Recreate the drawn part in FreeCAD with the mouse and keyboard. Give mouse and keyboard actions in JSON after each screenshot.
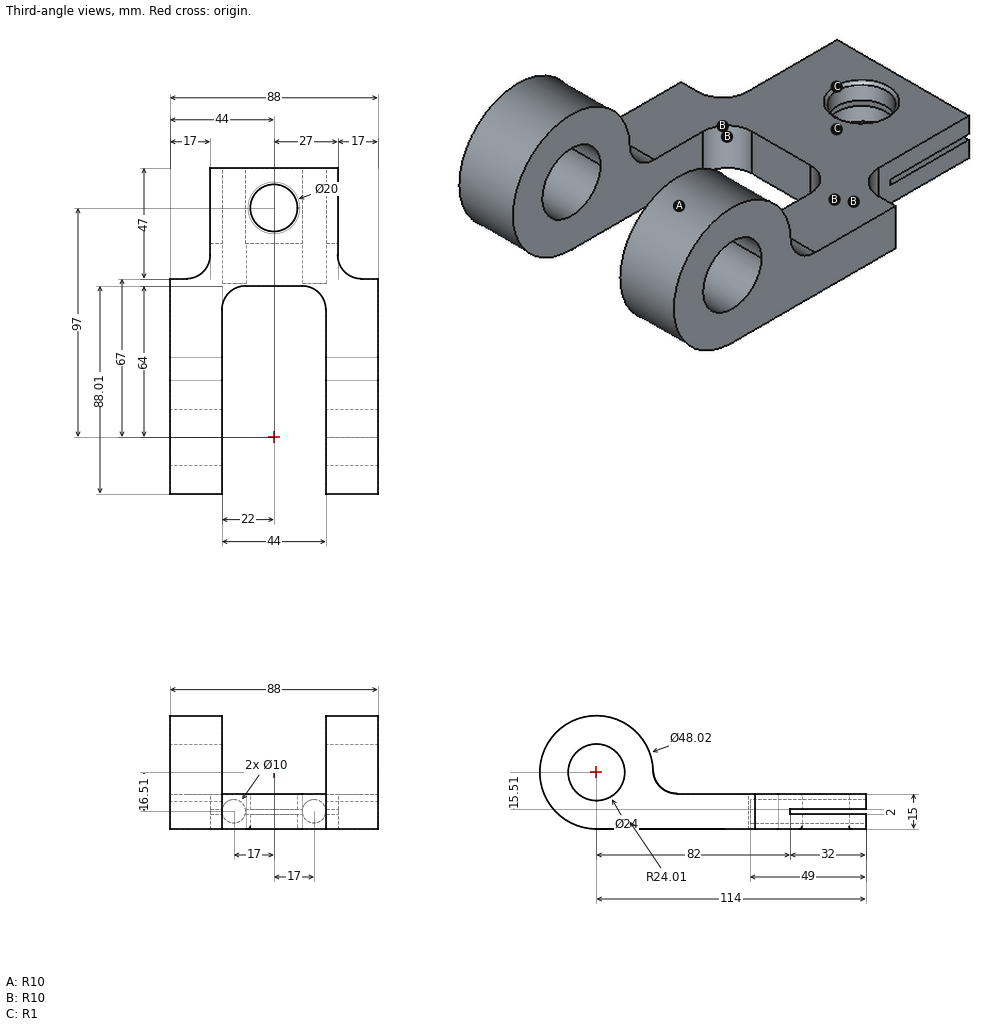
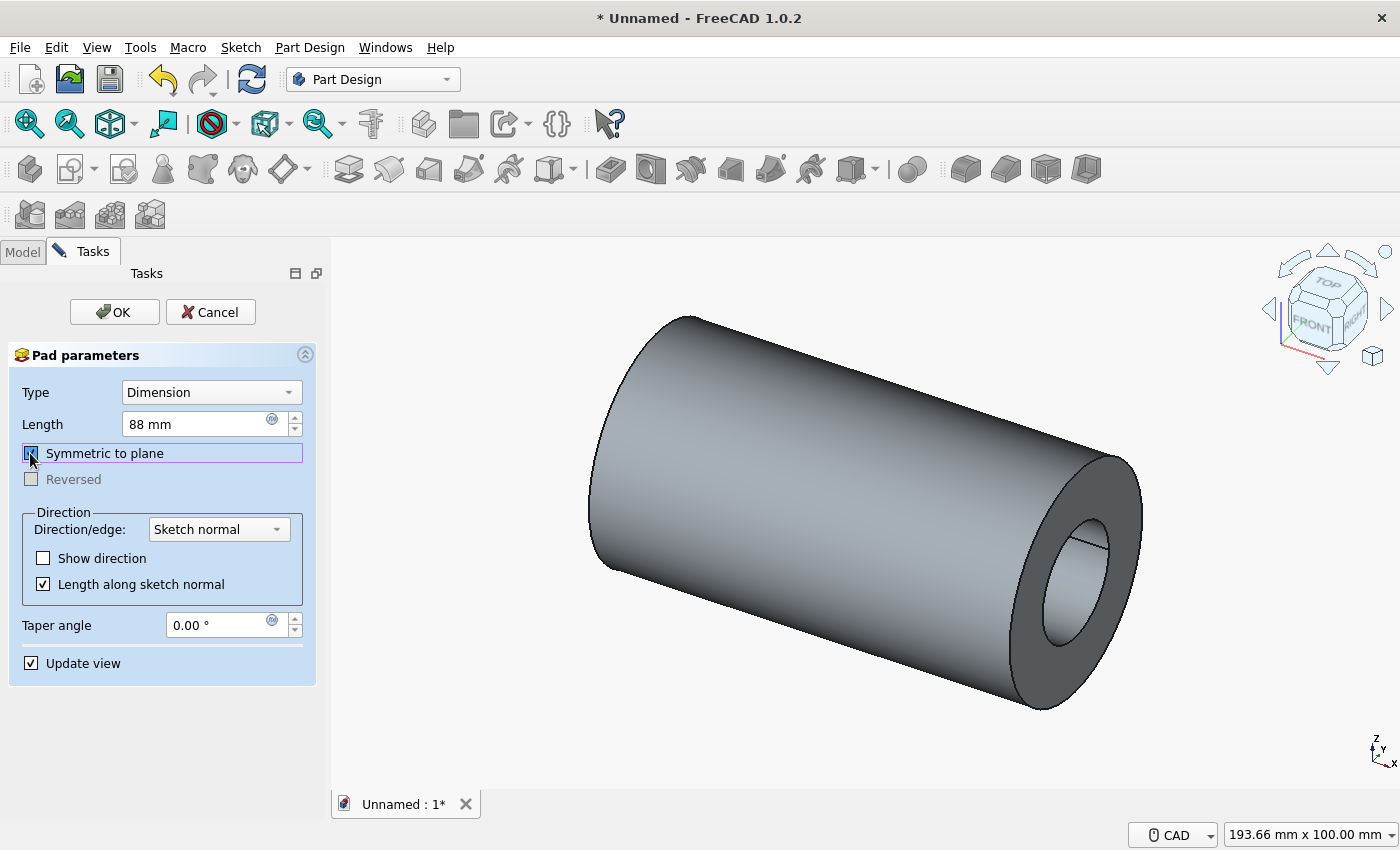
{"action": "left_click", "coordinate": [115, 312]}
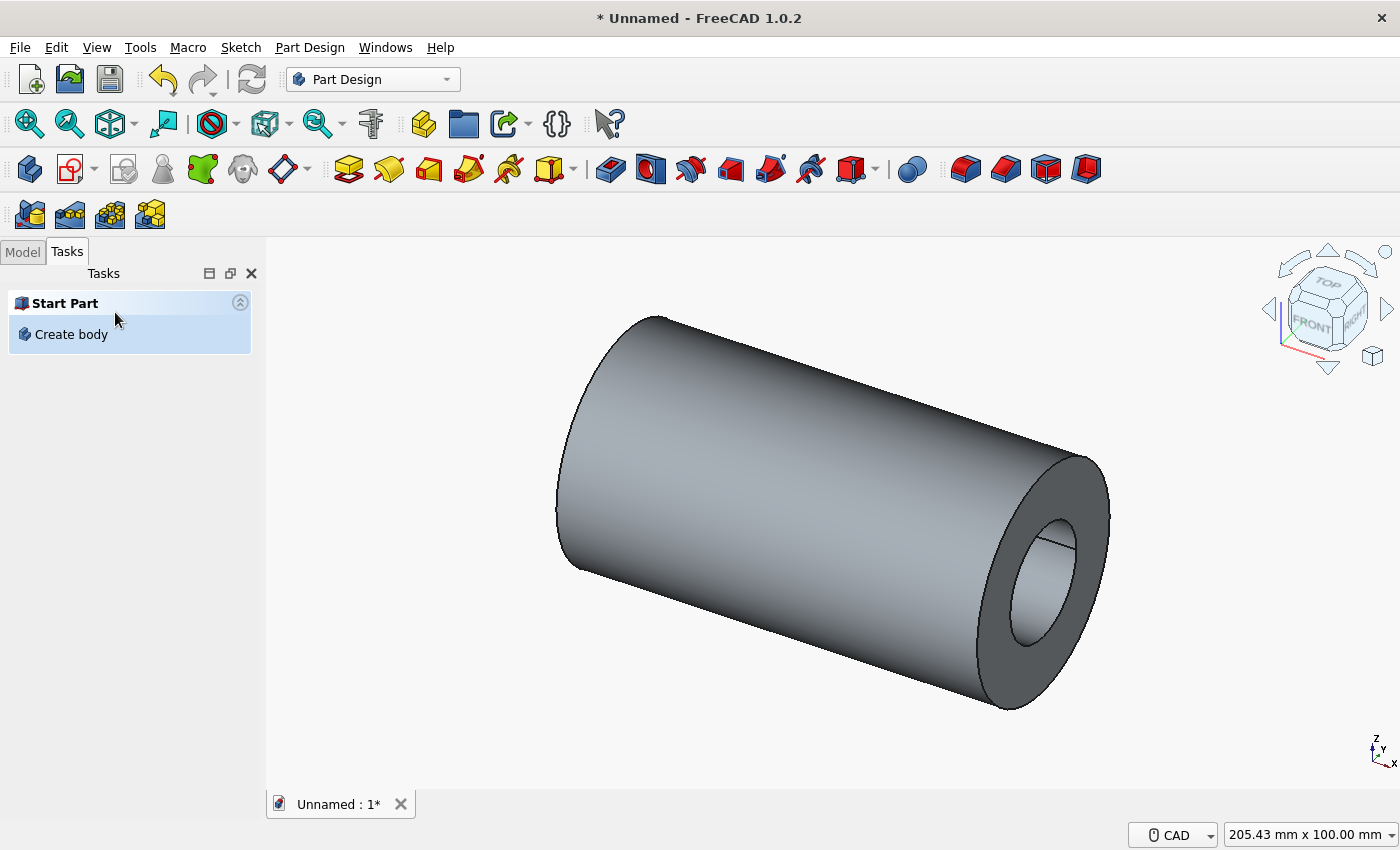
{"action": "left_click", "coordinate": [70, 170]}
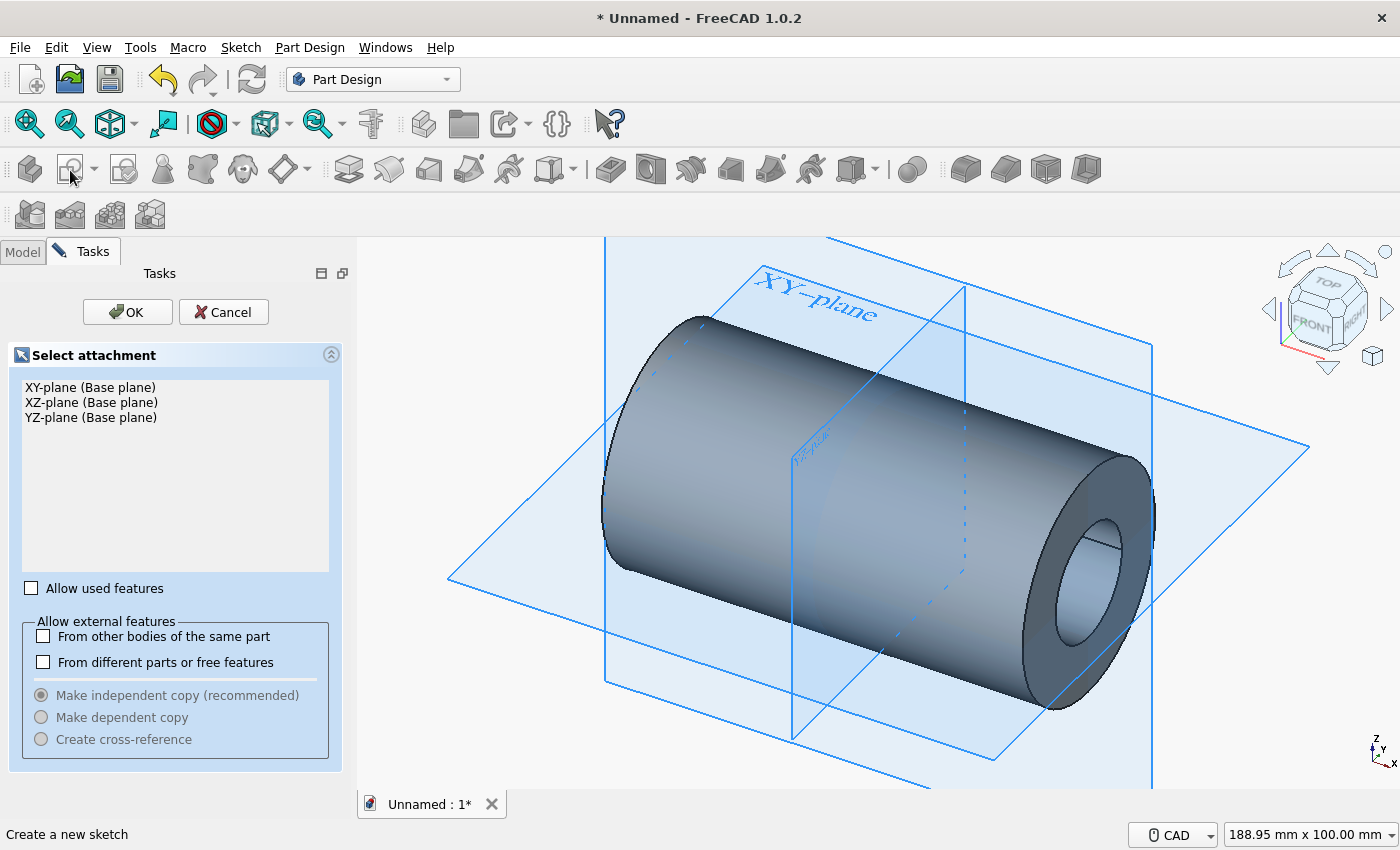
{"action": "left_click", "coordinate": [82, 418]}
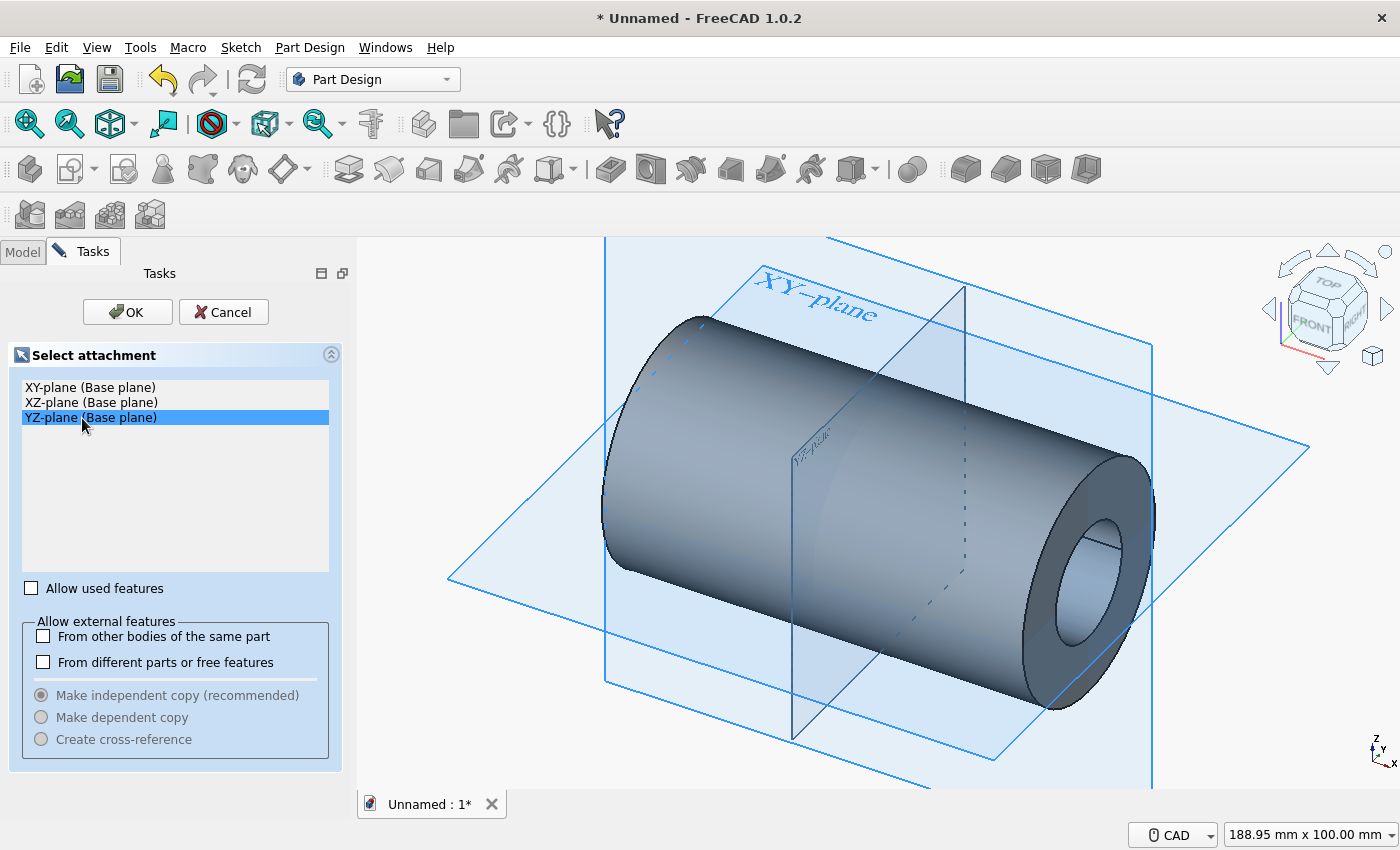
{"action": "left_click", "coordinate": [128, 312]}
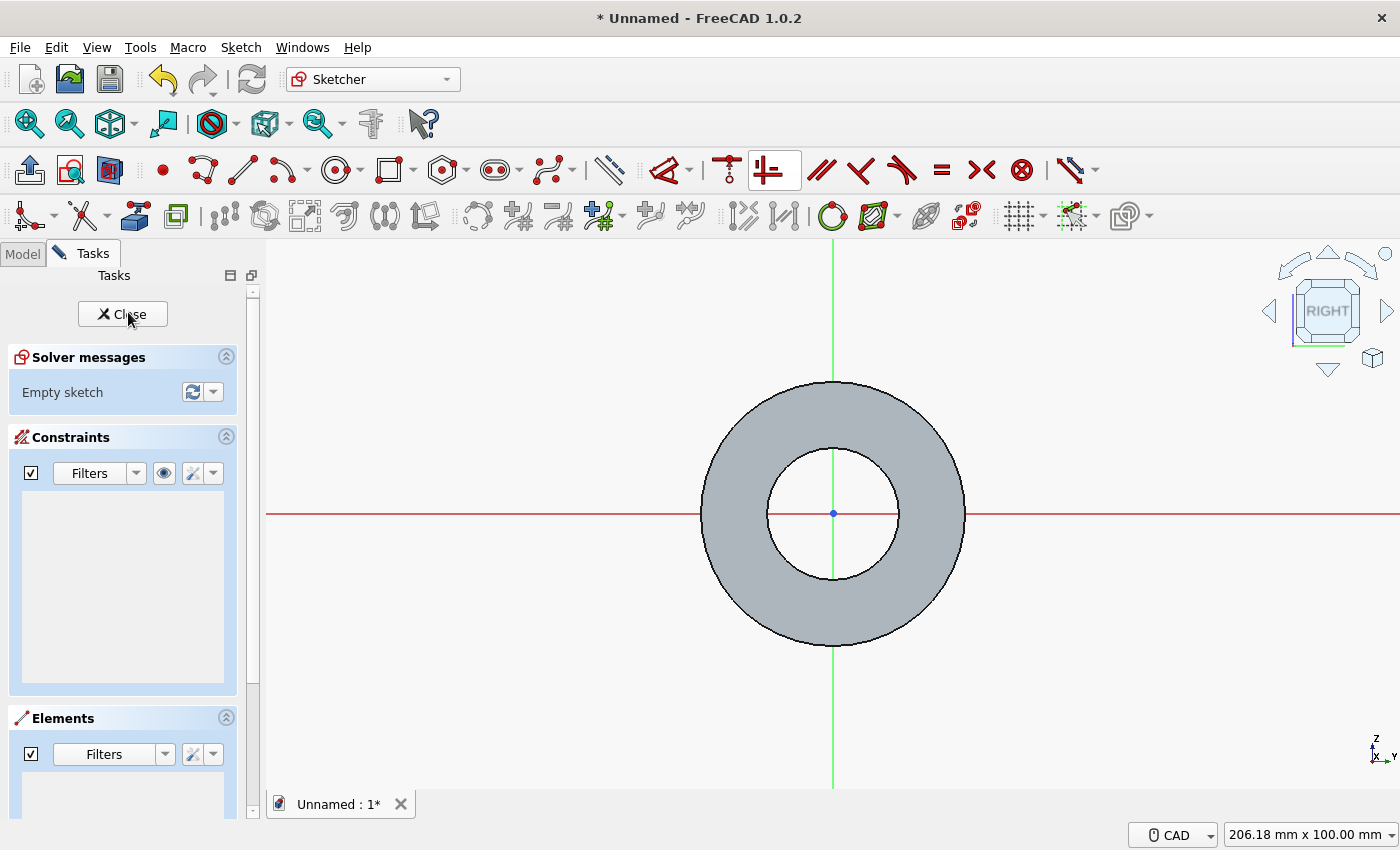
{"action": "left_click", "coordinate": [110, 170]}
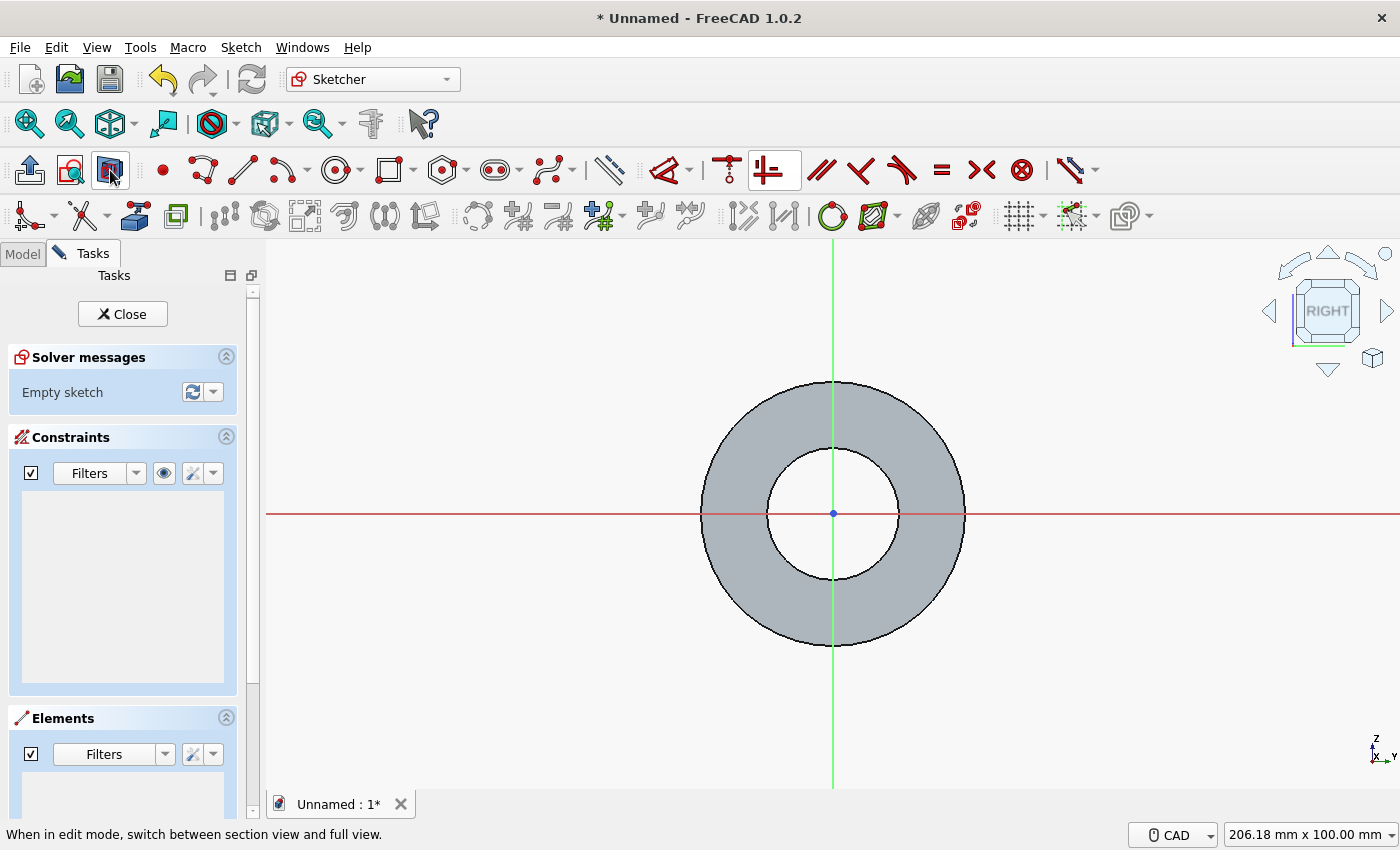
{"action": "scroll", "coordinate": [294, 380], "scroll_direction": "down", "scroll_amount": 2}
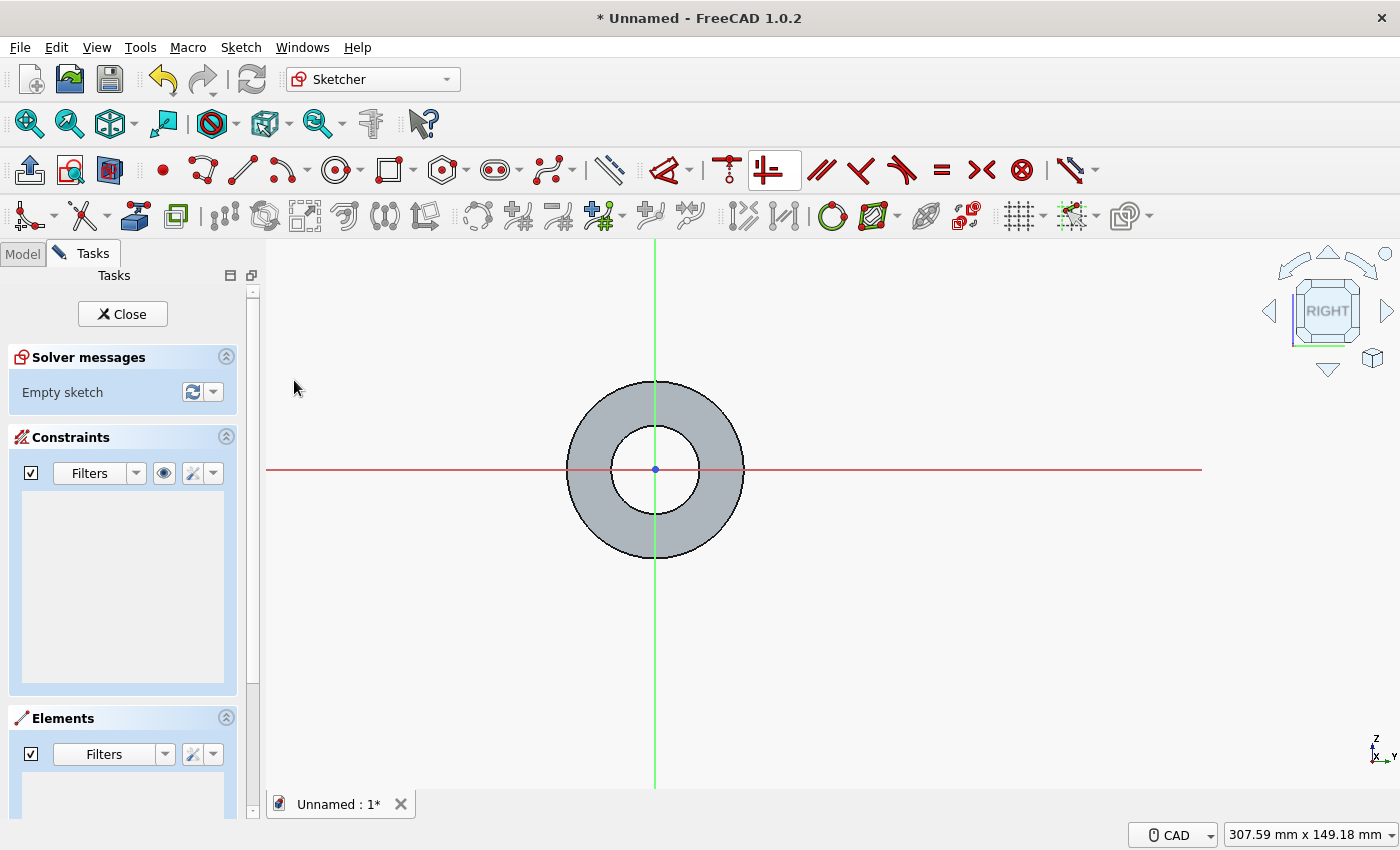
{"action": "scroll", "coordinate": [1071, 515], "scroll_direction": "up", "scroll_amount": 2}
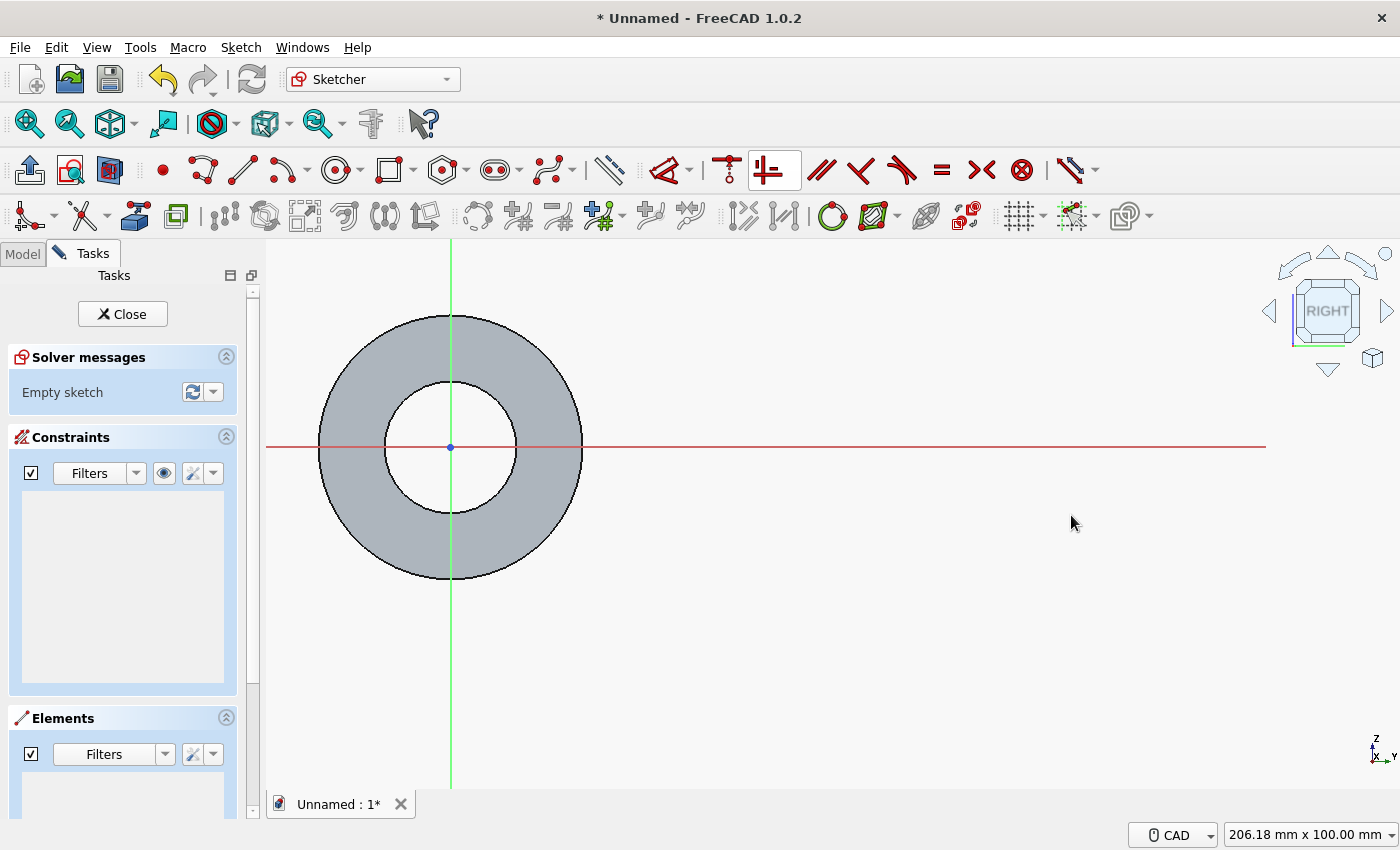
{"action": "left_click", "coordinate": [204, 170]}